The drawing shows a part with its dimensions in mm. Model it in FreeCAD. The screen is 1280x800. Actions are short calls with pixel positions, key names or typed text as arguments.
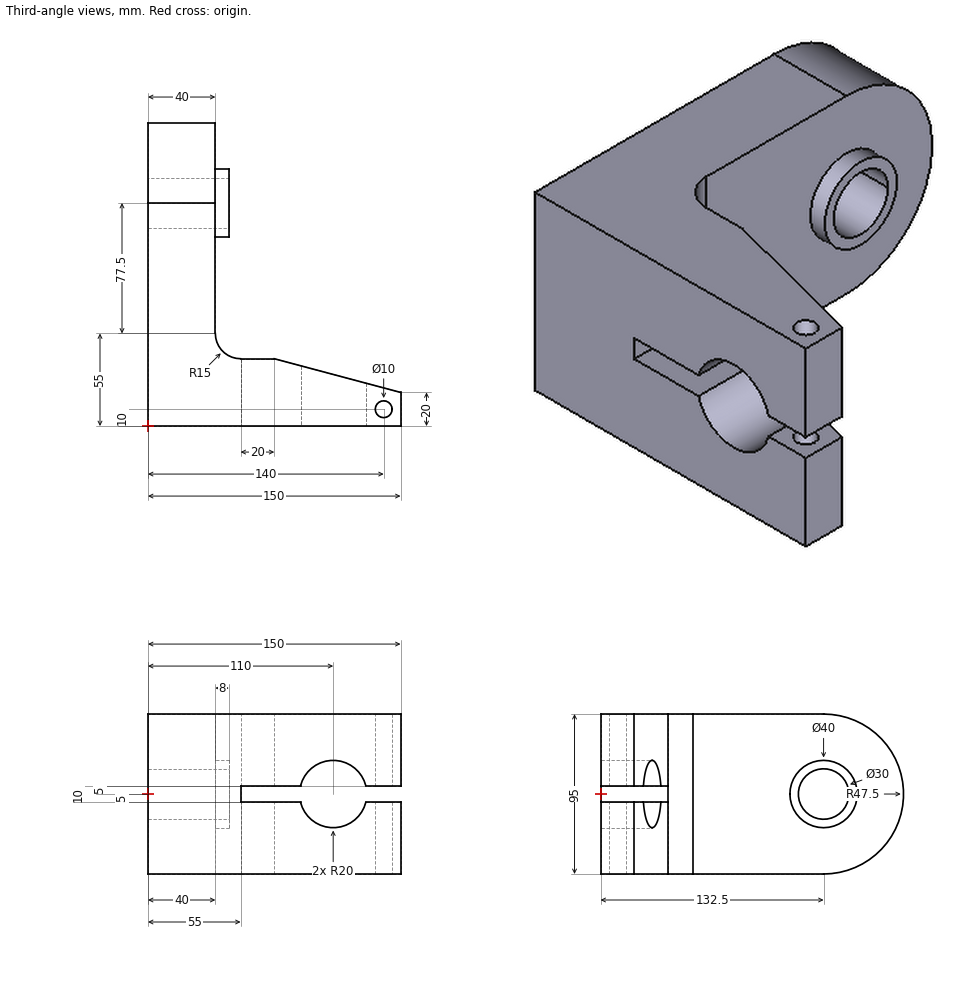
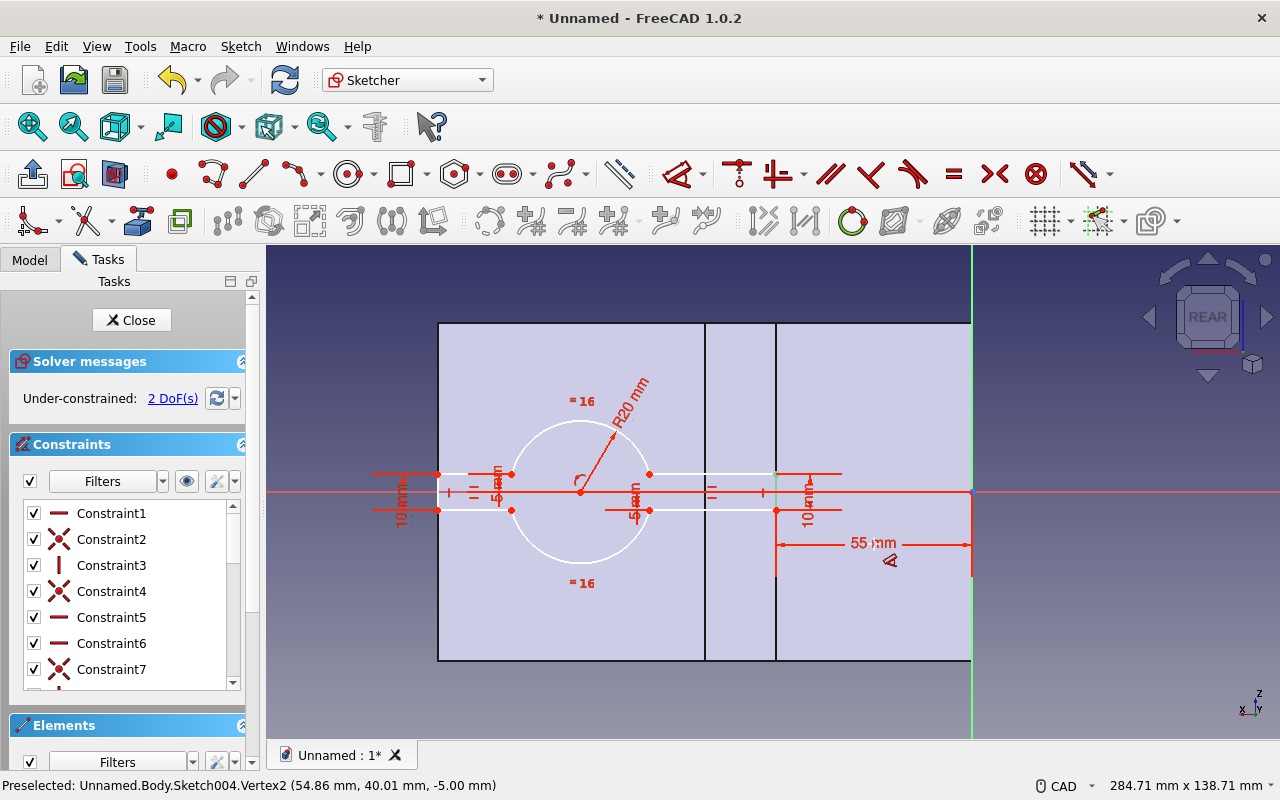
click(438, 474)
click(705, 440)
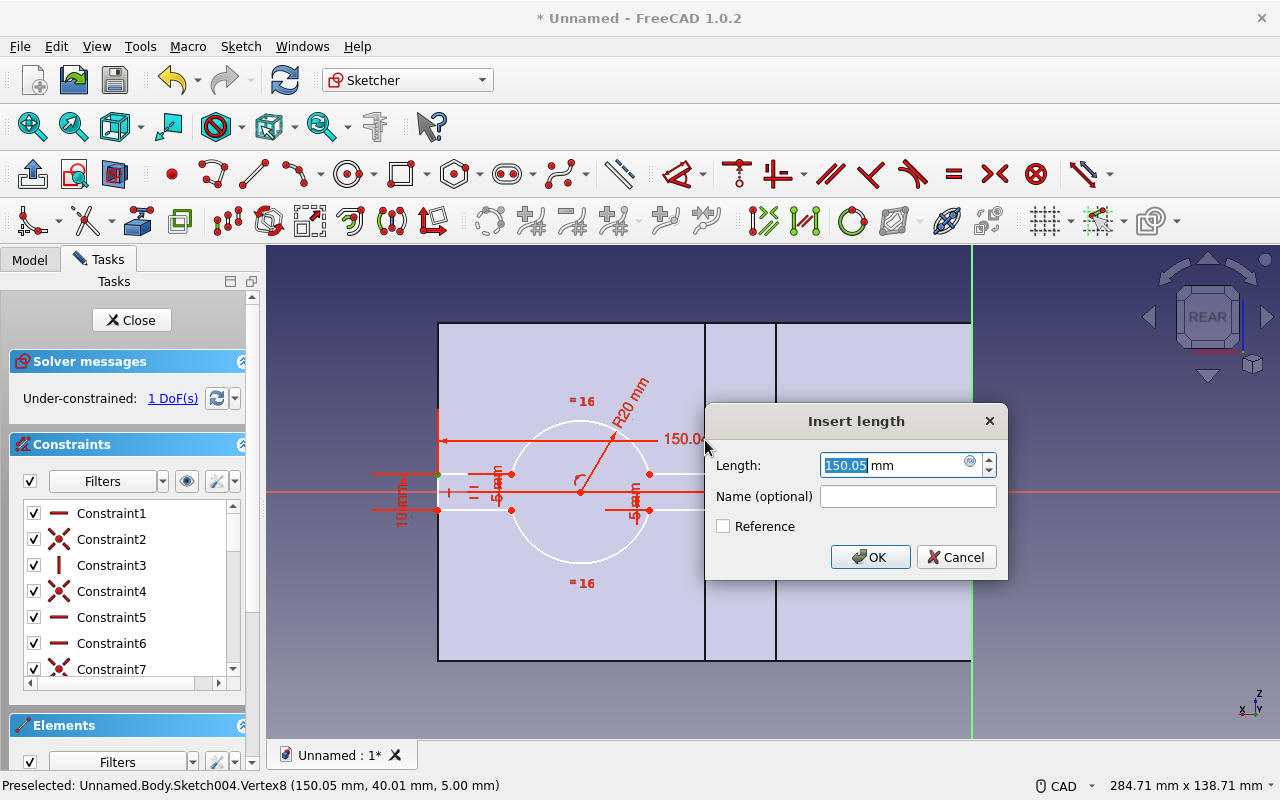
text(150)
key(Return)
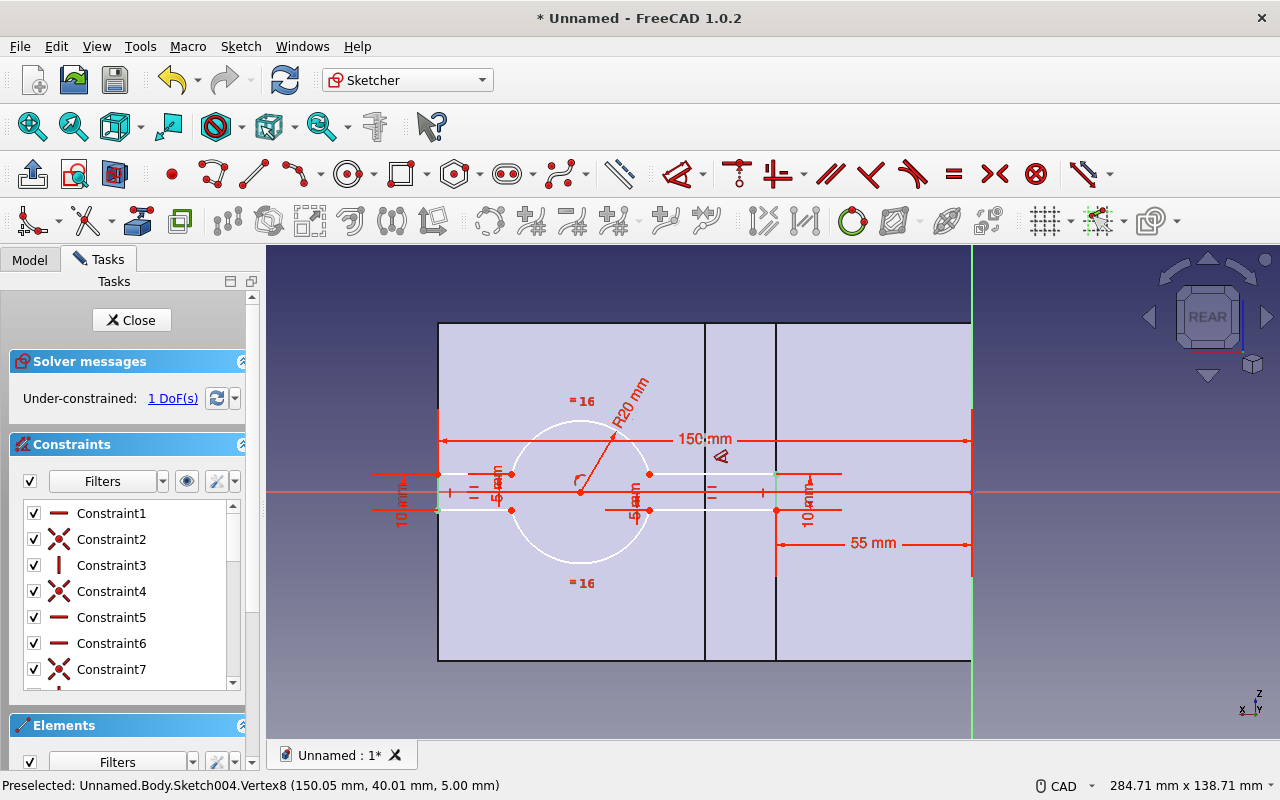
click(581, 492)
click(776, 526)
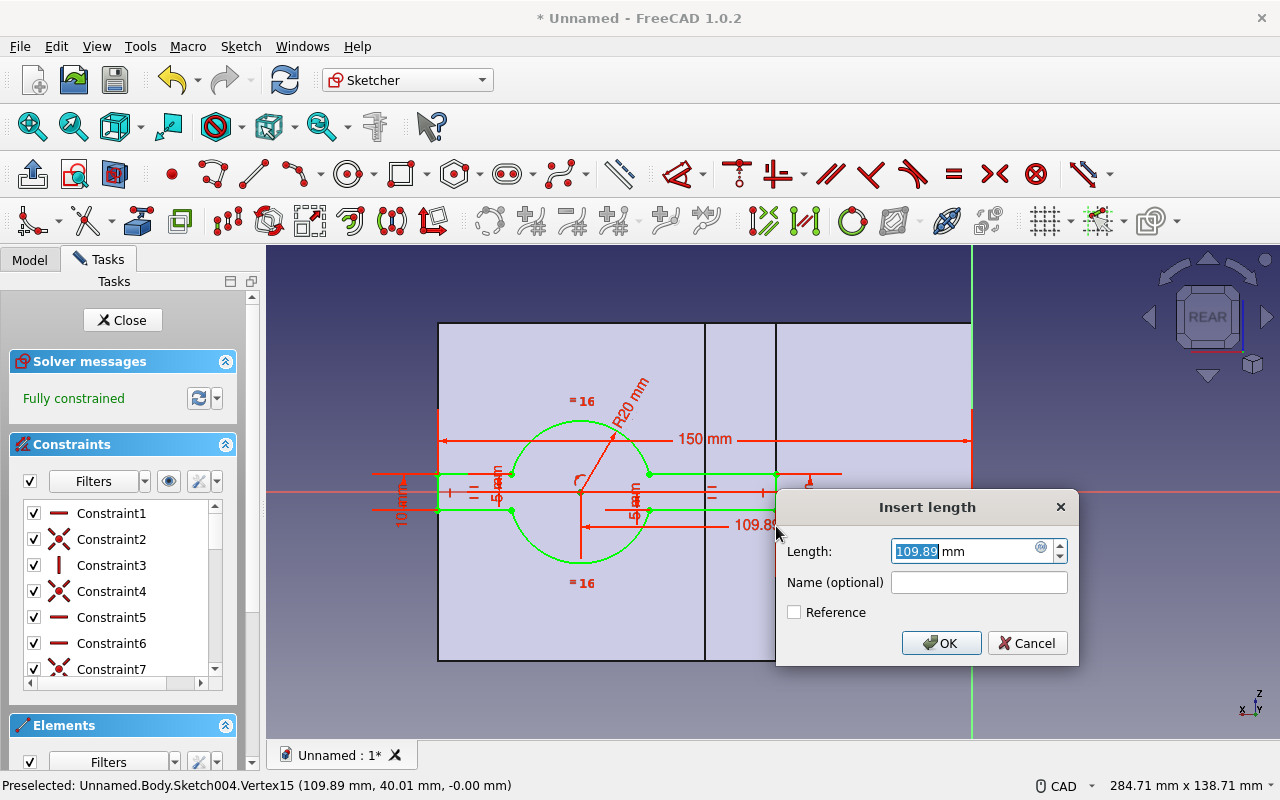
text(110)
key(Return)
key(Escape)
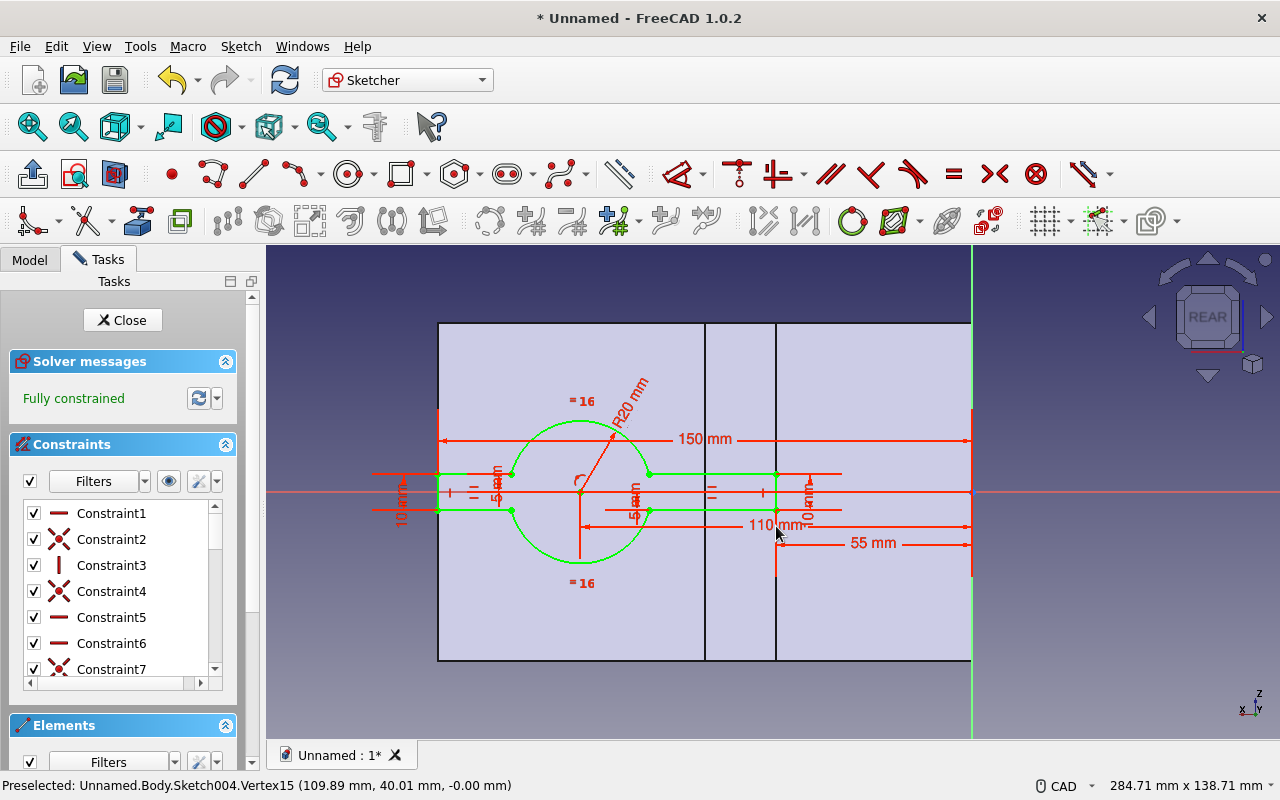
click(123, 320)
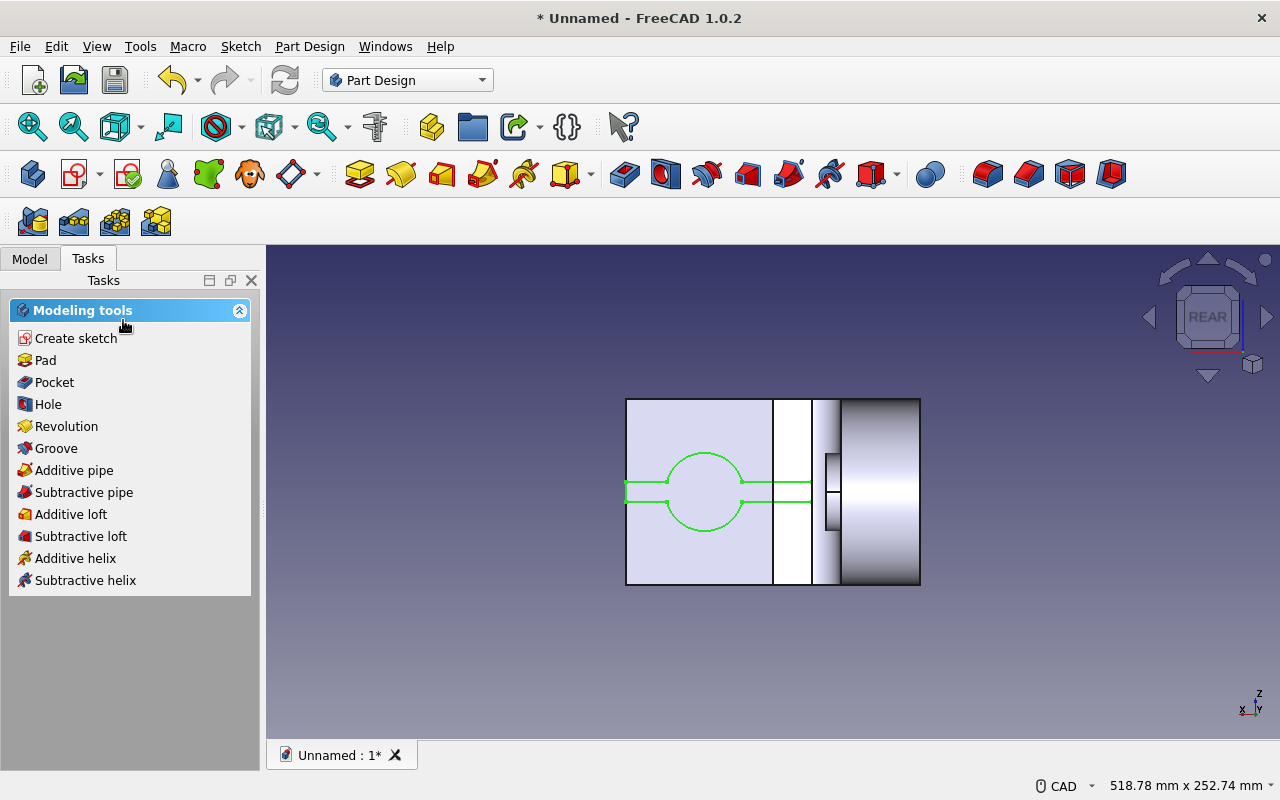
click(625, 174)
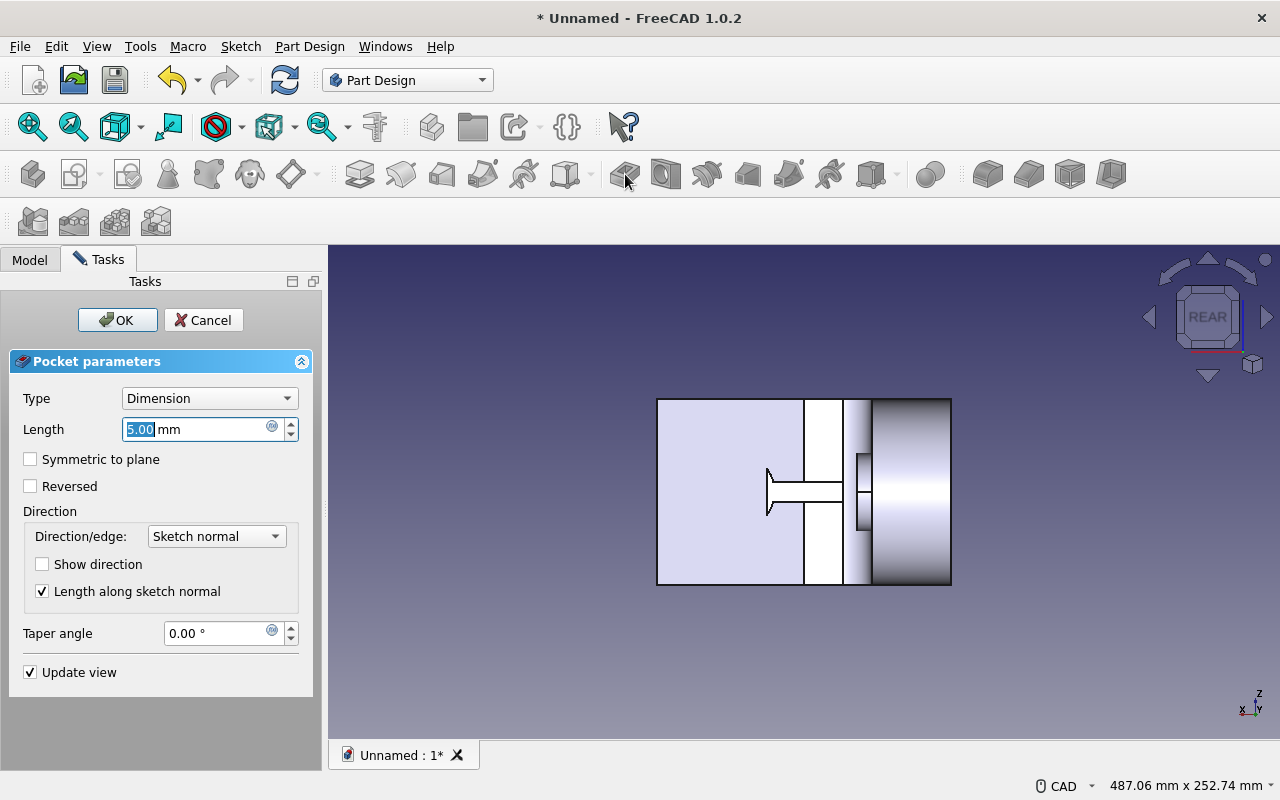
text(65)
key(Tab)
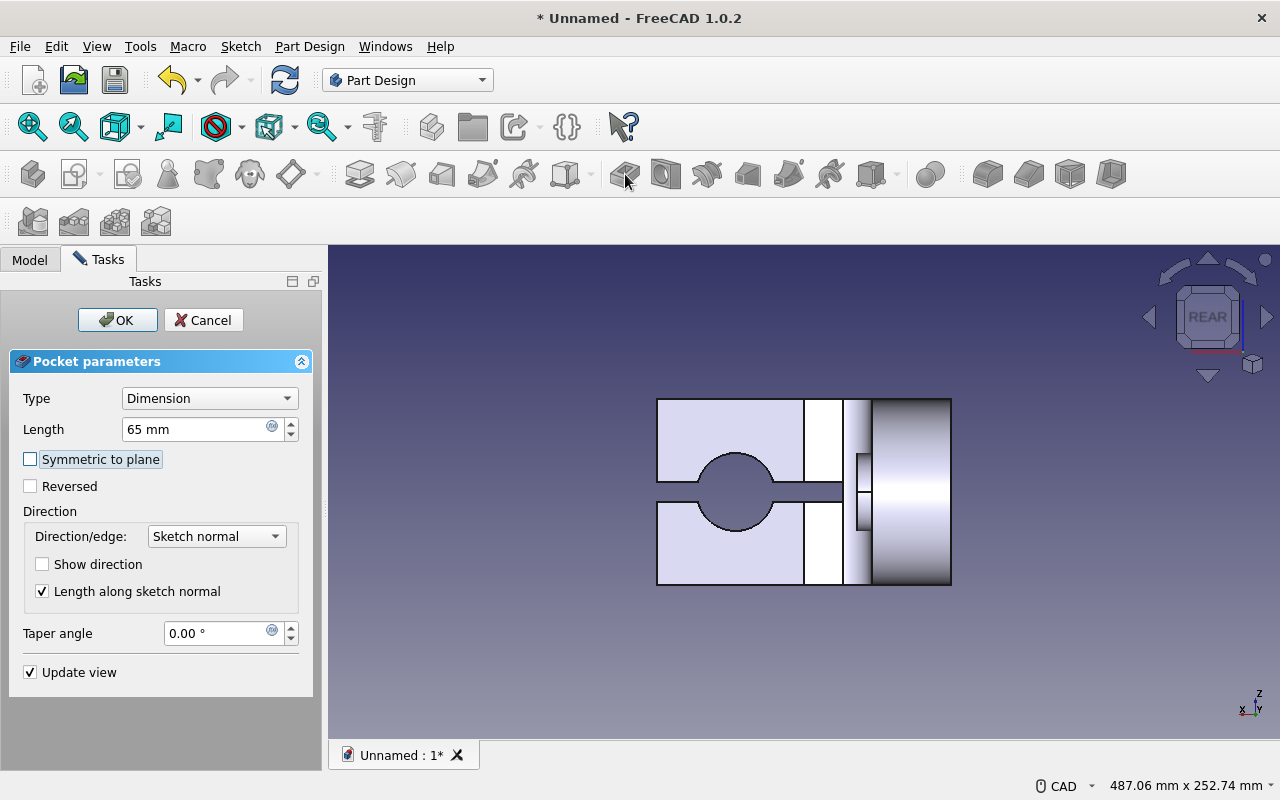
click(118, 320)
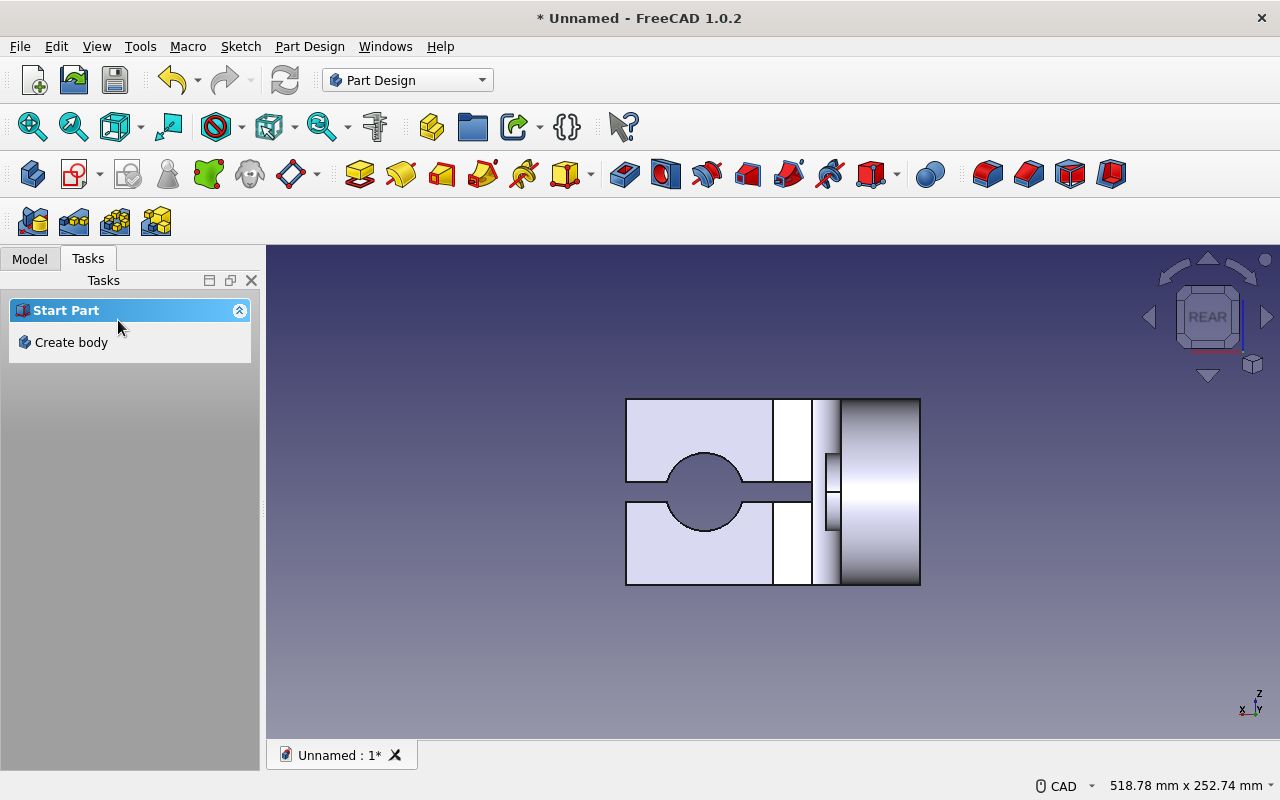
click(33, 128)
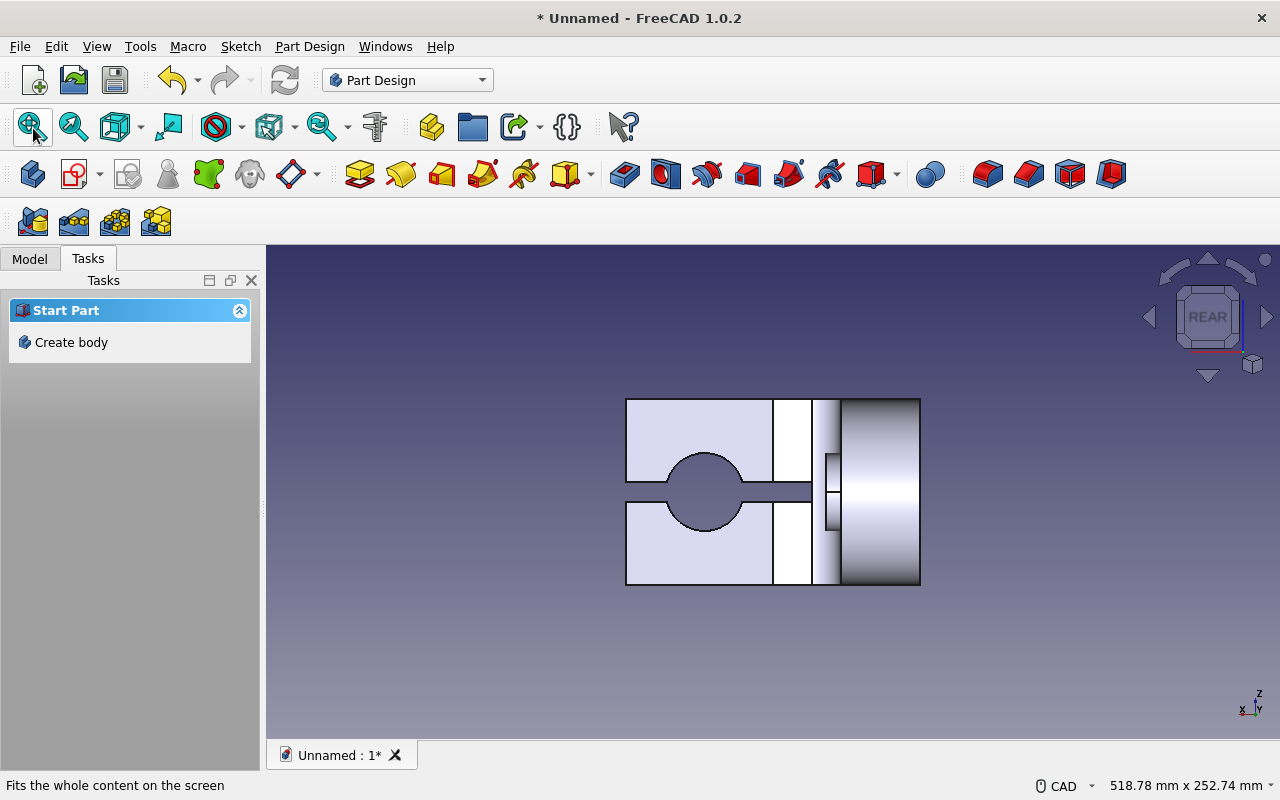
key(0)